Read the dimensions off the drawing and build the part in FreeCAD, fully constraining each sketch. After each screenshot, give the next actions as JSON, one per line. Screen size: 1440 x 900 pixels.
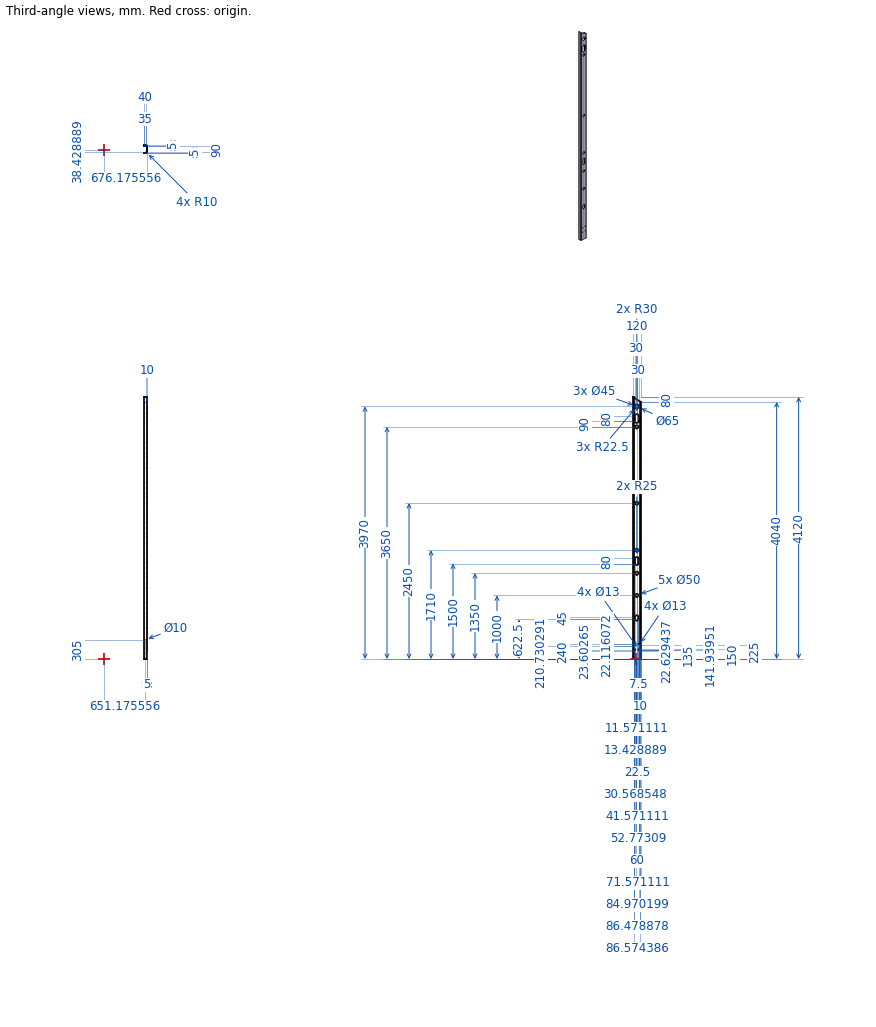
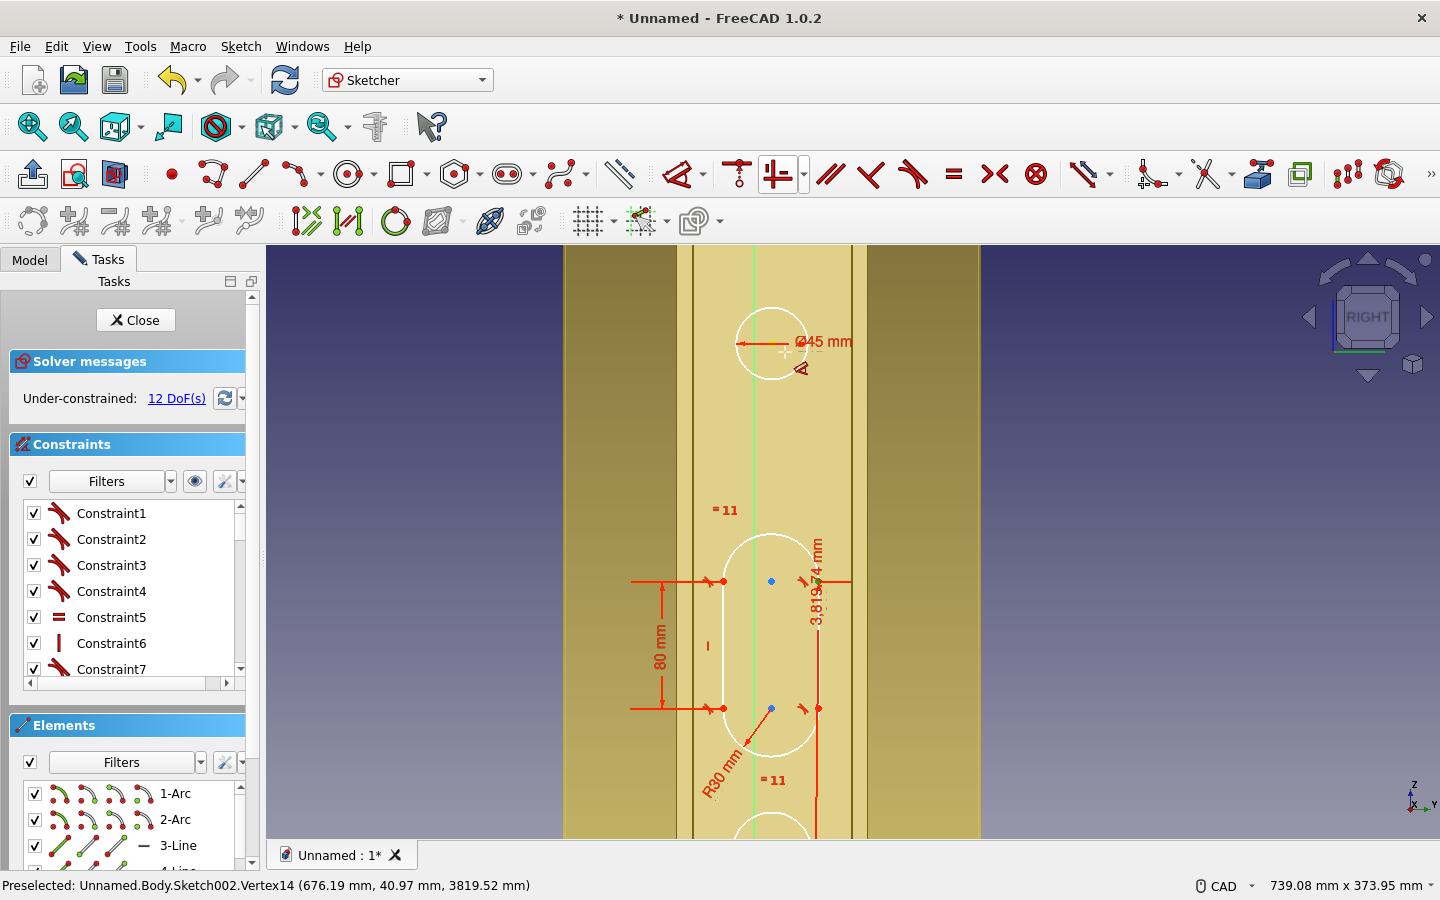
{"action": "left_click", "coordinate": [772, 344]}
{"action": "left_click", "coordinate": [812, 310]}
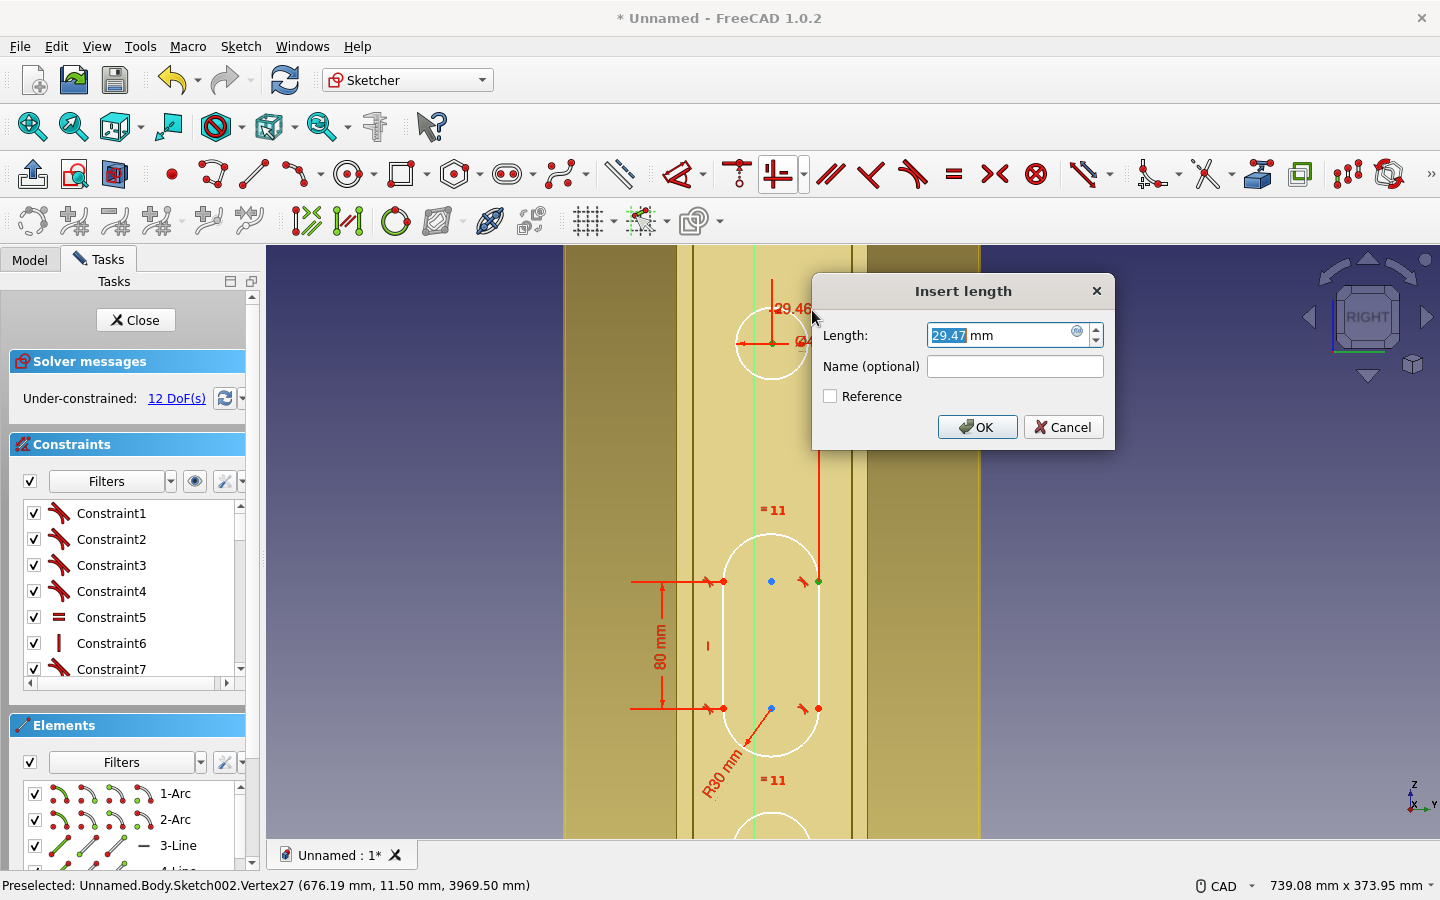
{"action": "type", "text": "30"}
{"action": "key", "text": "Return"}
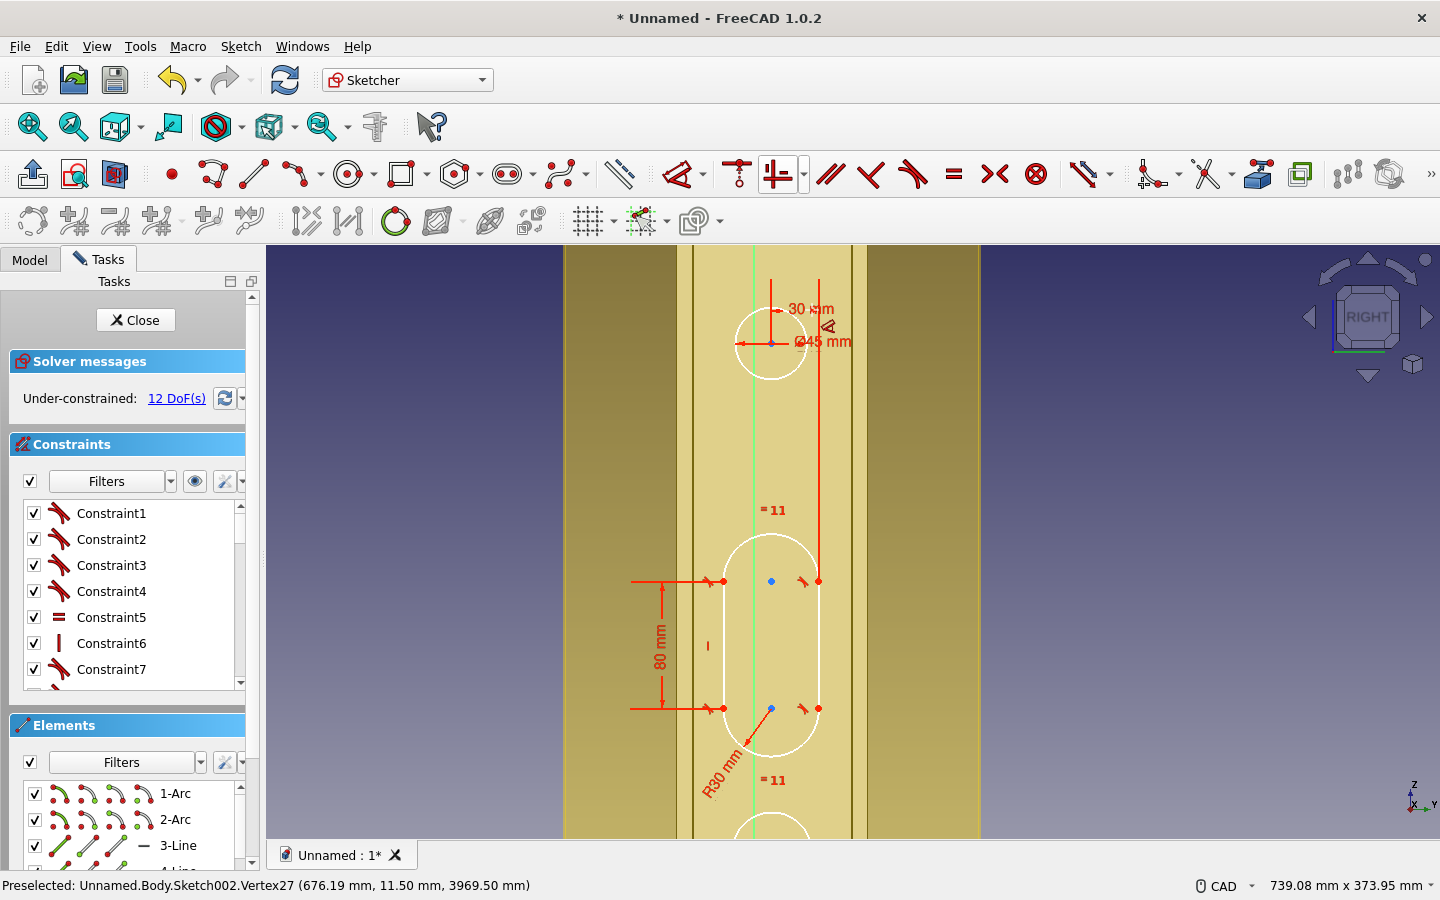
{"action": "left_click", "coordinate": [724, 709]}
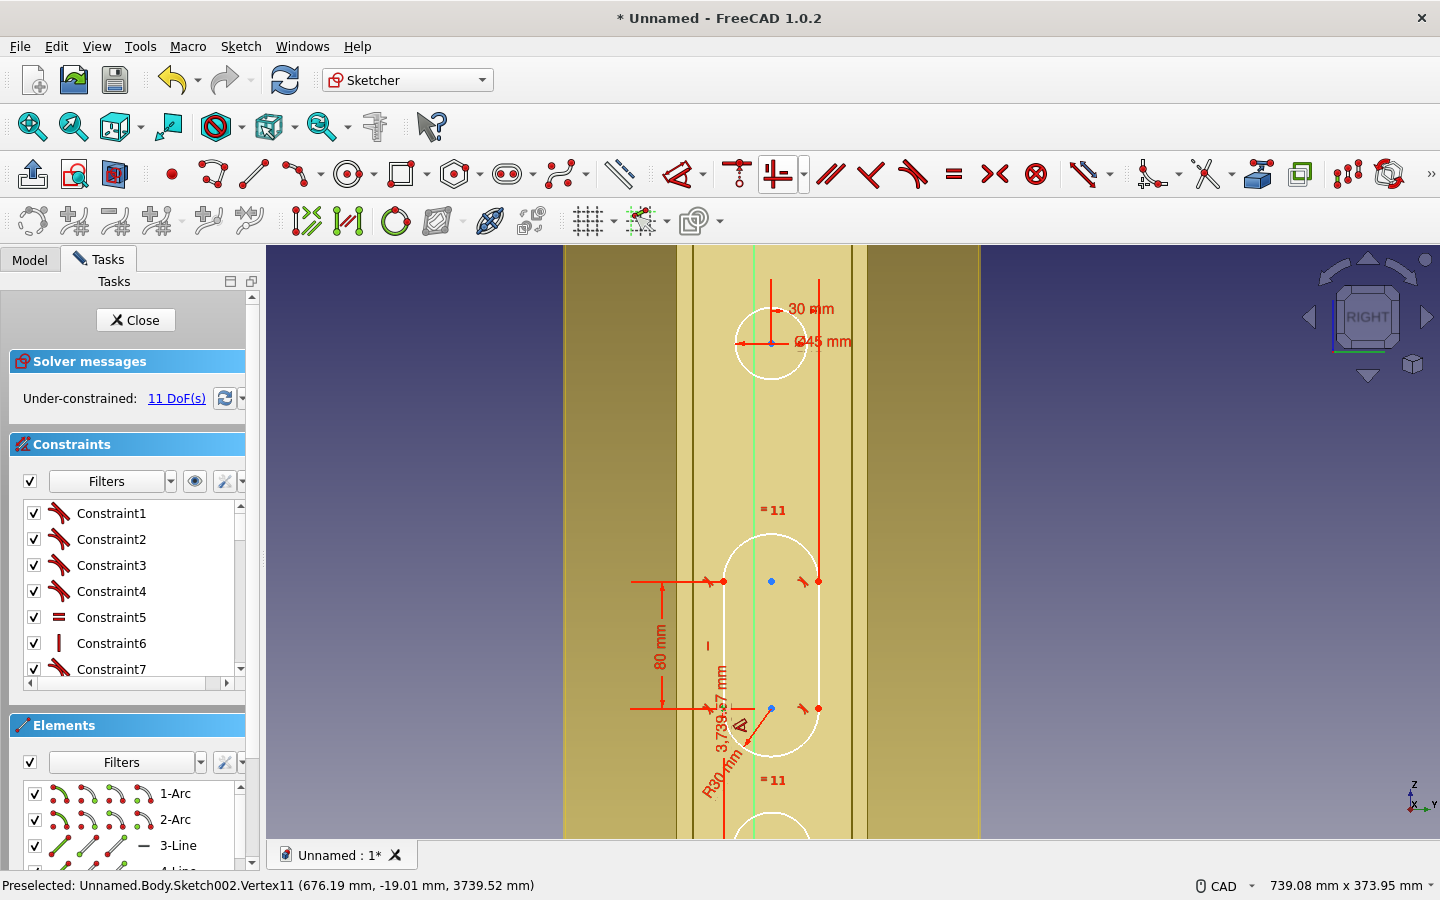
{"action": "scroll", "coordinate": [785, 352], "scroll_direction": "down", "scroll_amount": 14}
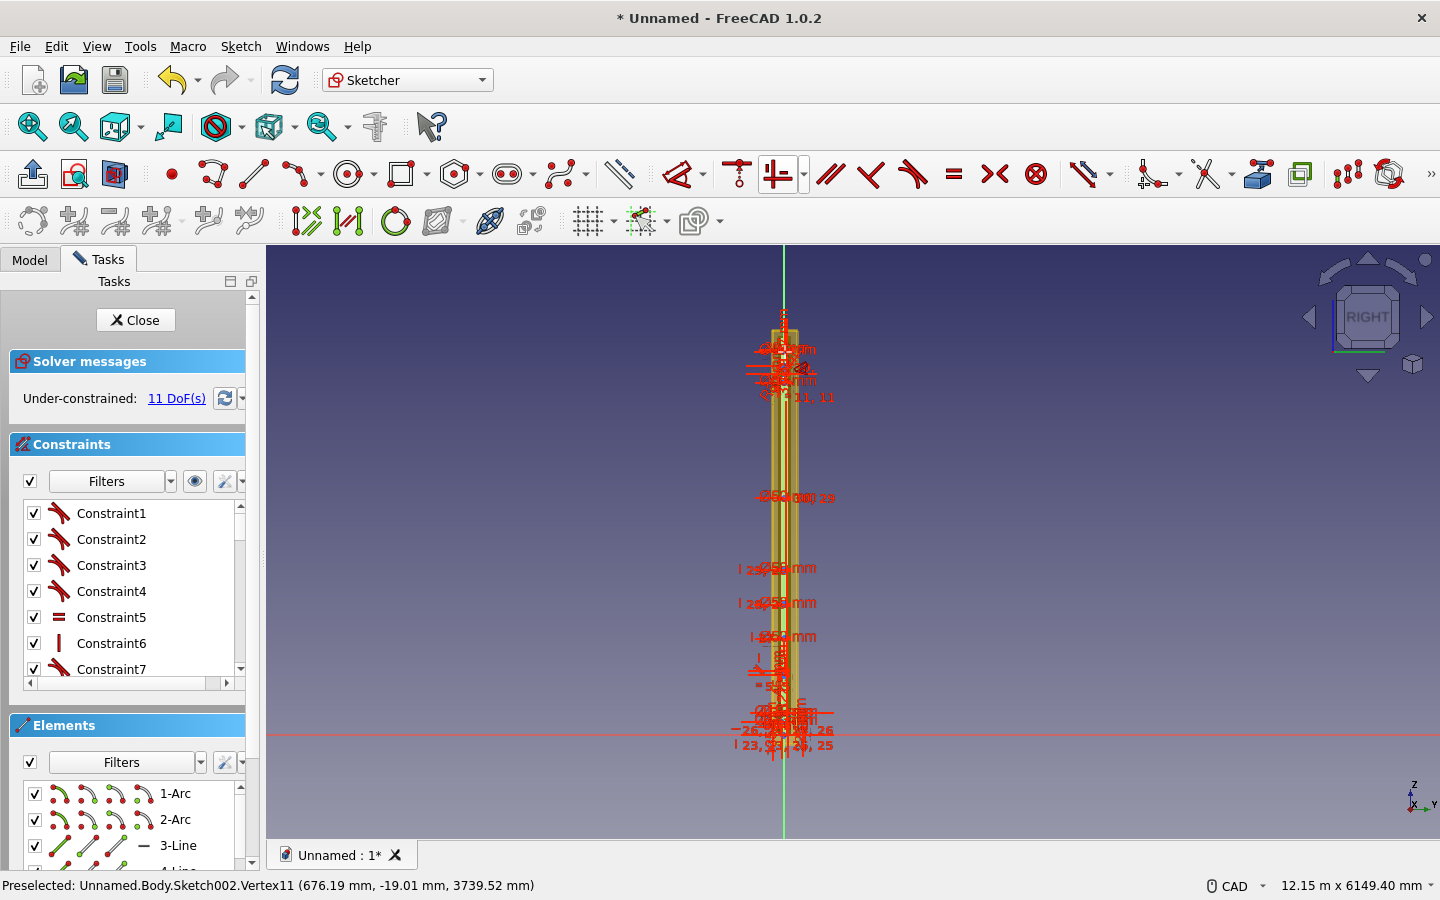
{"action": "scroll", "coordinate": [785, 383], "scroll_direction": "up", "scroll_amount": 14}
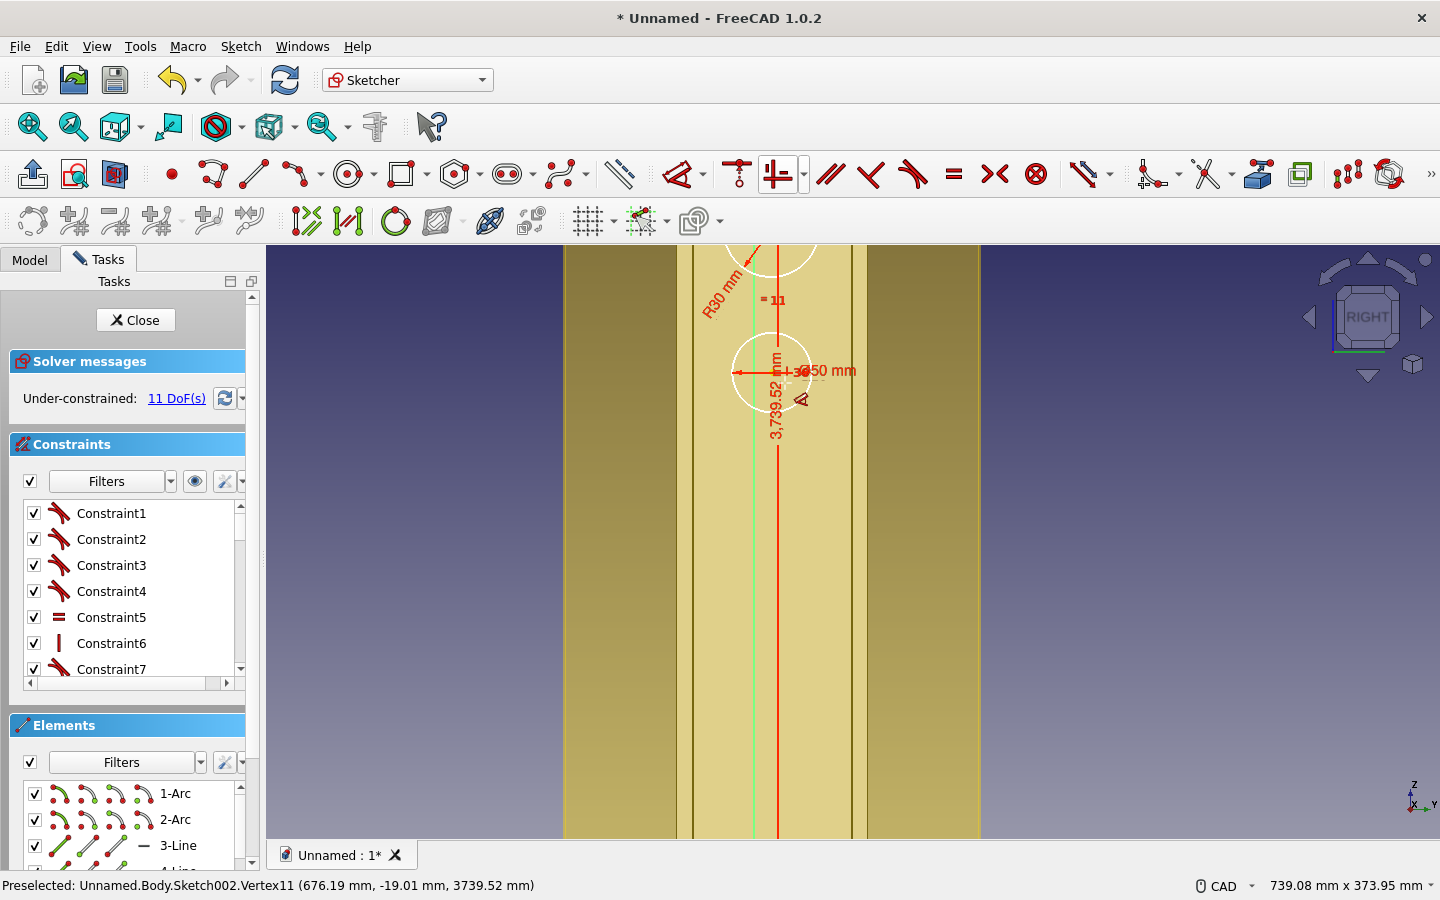
{"action": "left_click", "coordinate": [772, 373]}
{"action": "left_click", "coordinate": [731, 407]}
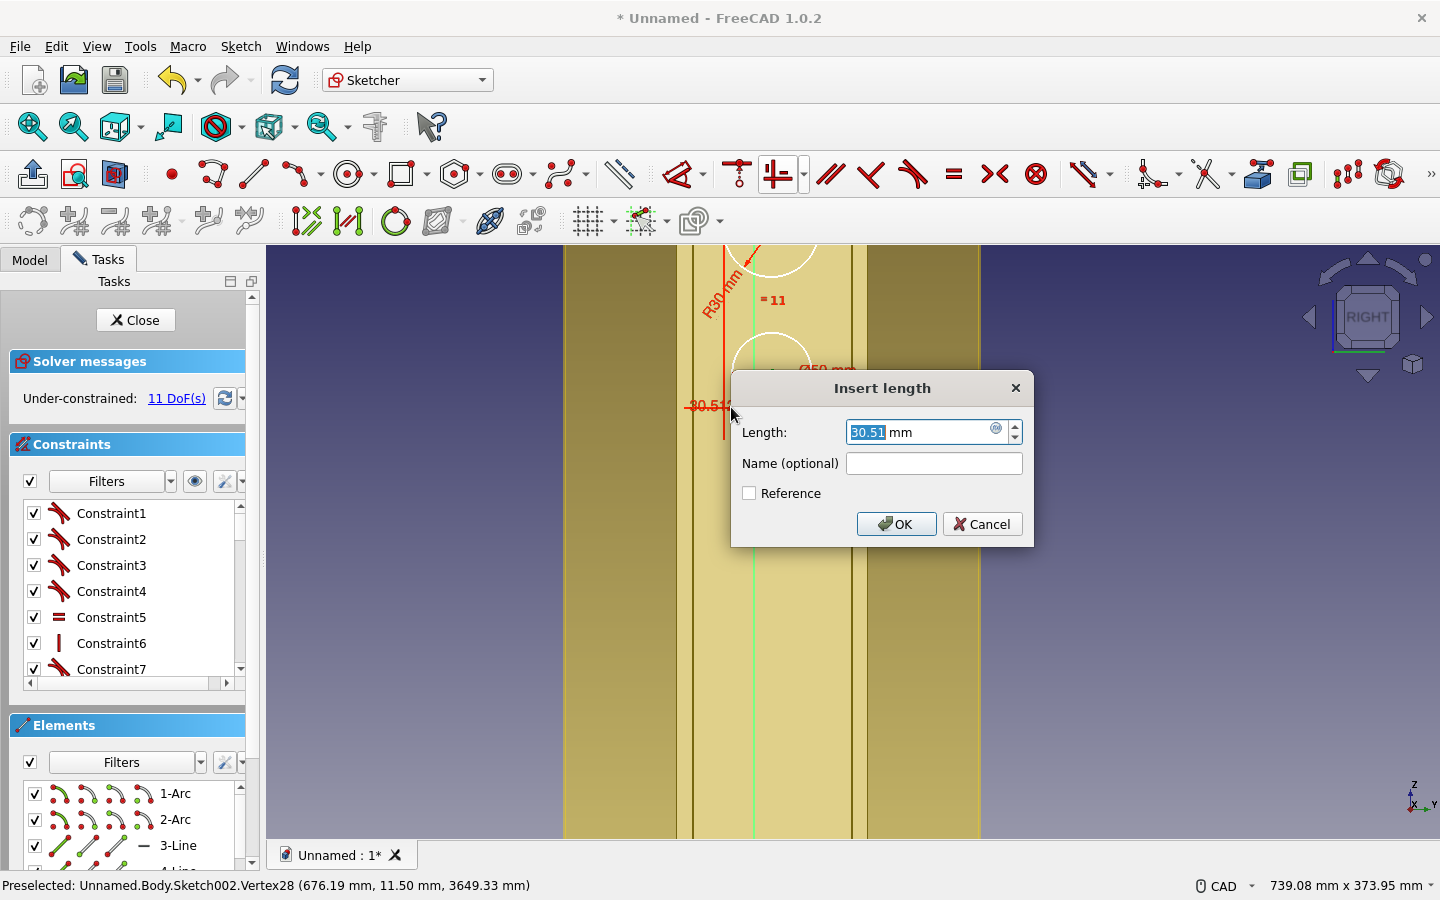
{"action": "type", "text": "30"}
{"action": "key", "text": "Return"}